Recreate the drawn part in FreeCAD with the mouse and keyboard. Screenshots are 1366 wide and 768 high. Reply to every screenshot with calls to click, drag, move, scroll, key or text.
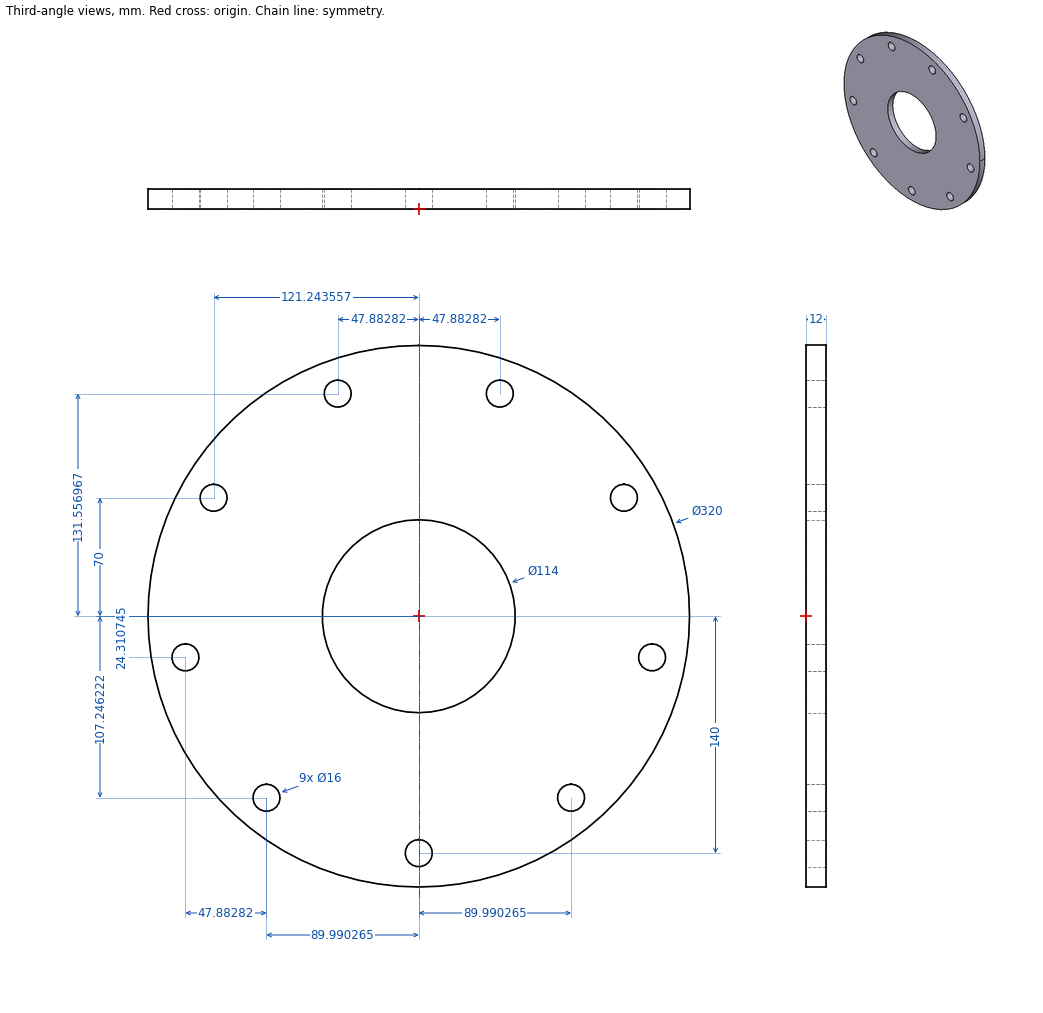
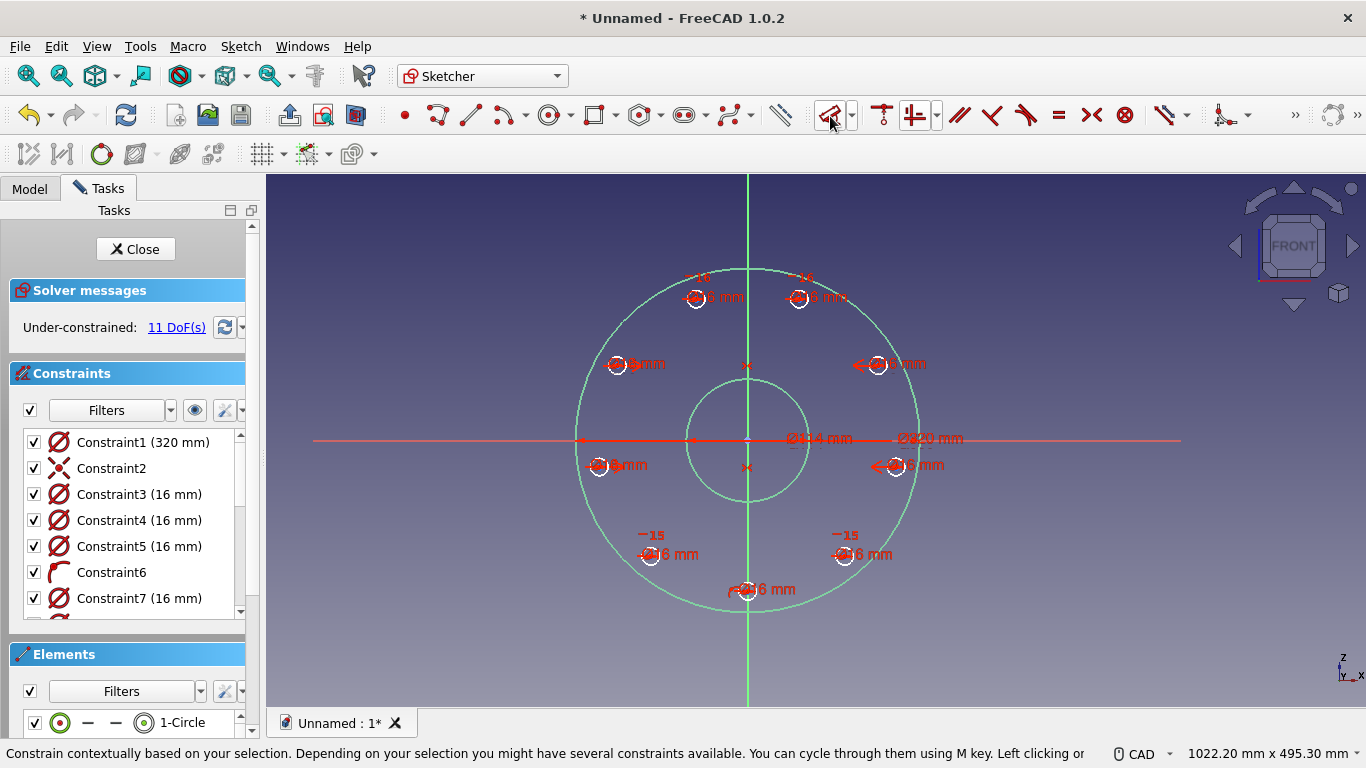
click(617, 366)
click(782, 420)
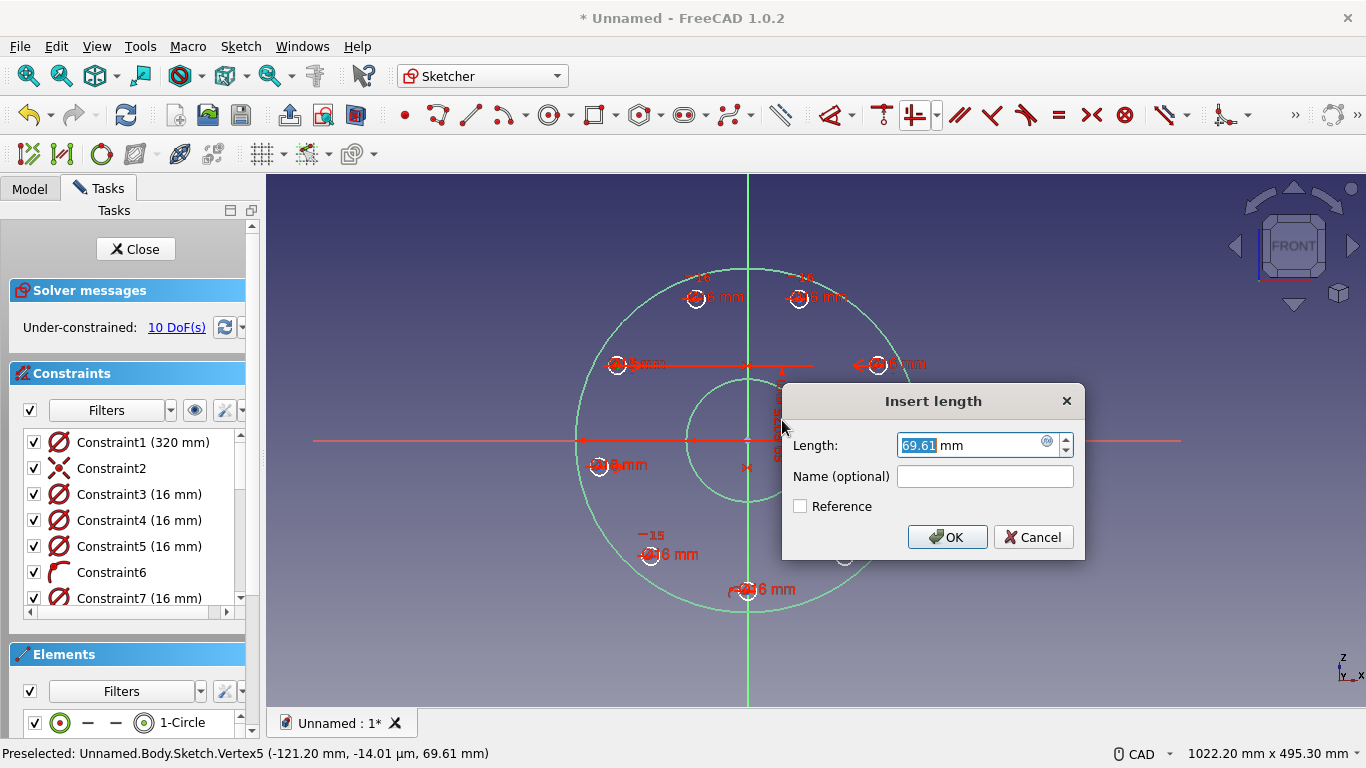
text(70)
key(Return)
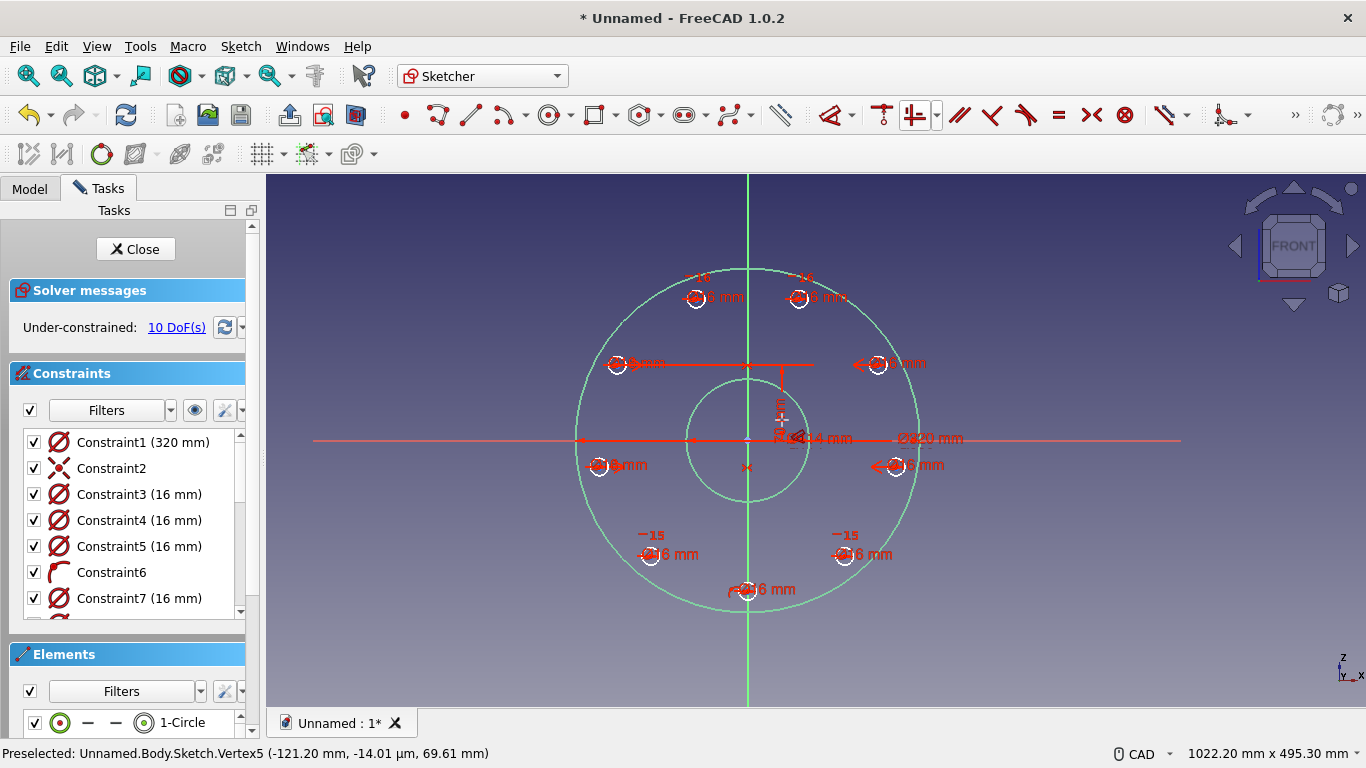
click(748, 591)
click(782, 516)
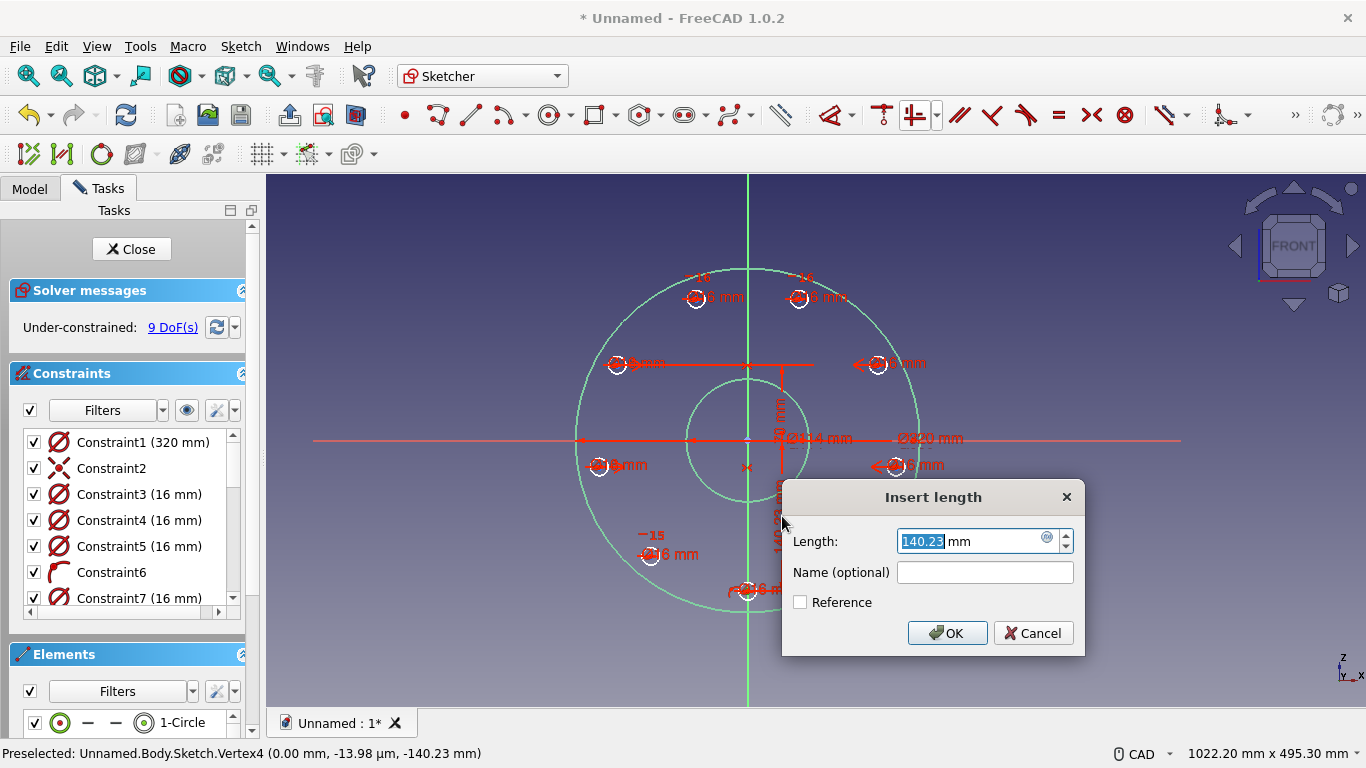
text(140)
key(Return)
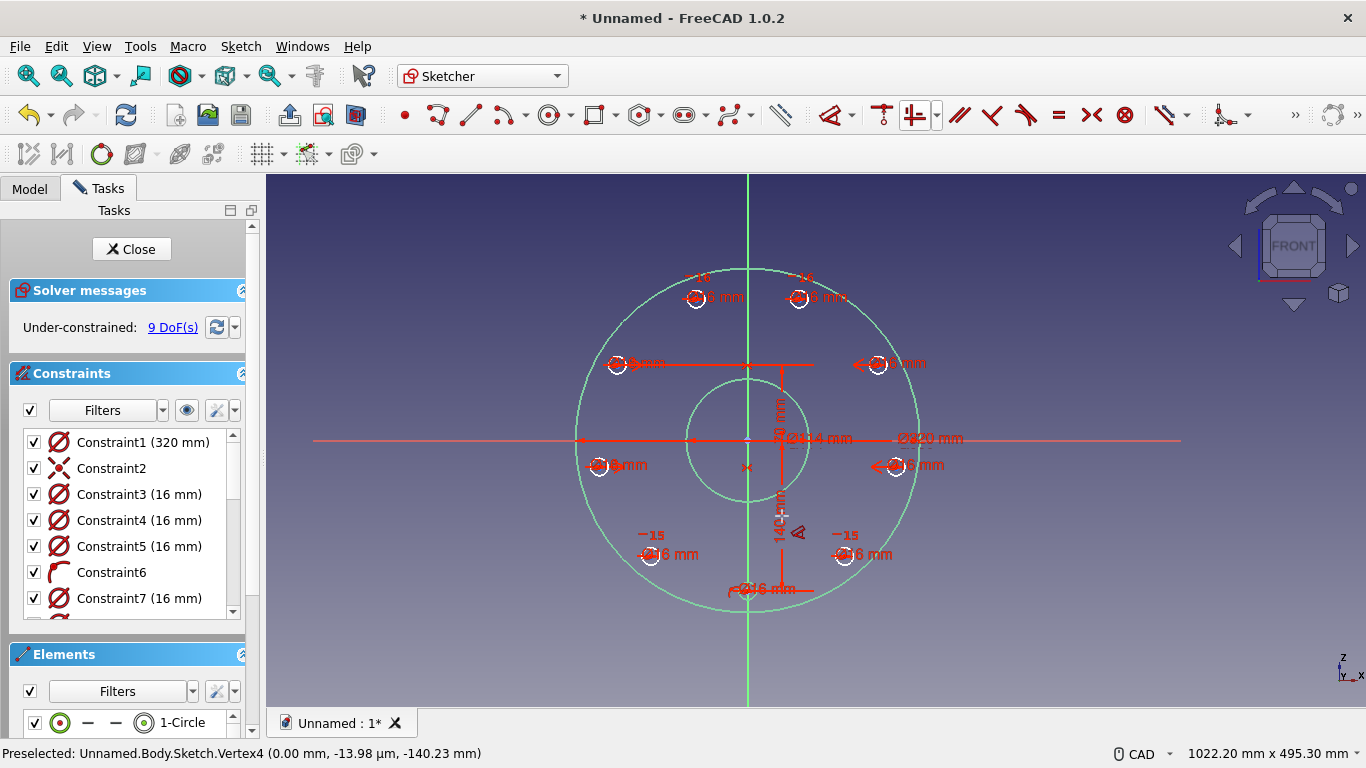
click(696, 299)
click(722, 474)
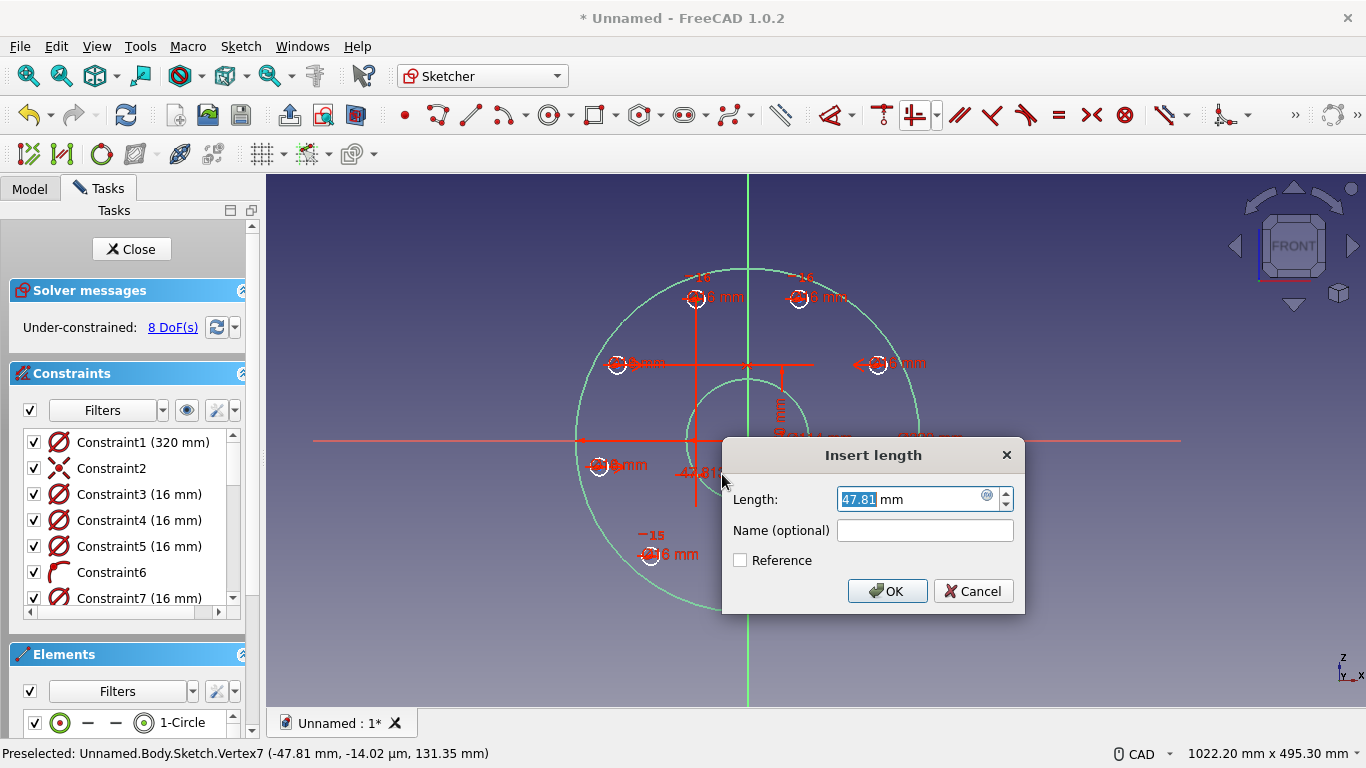
text(47.88282)
key(Return)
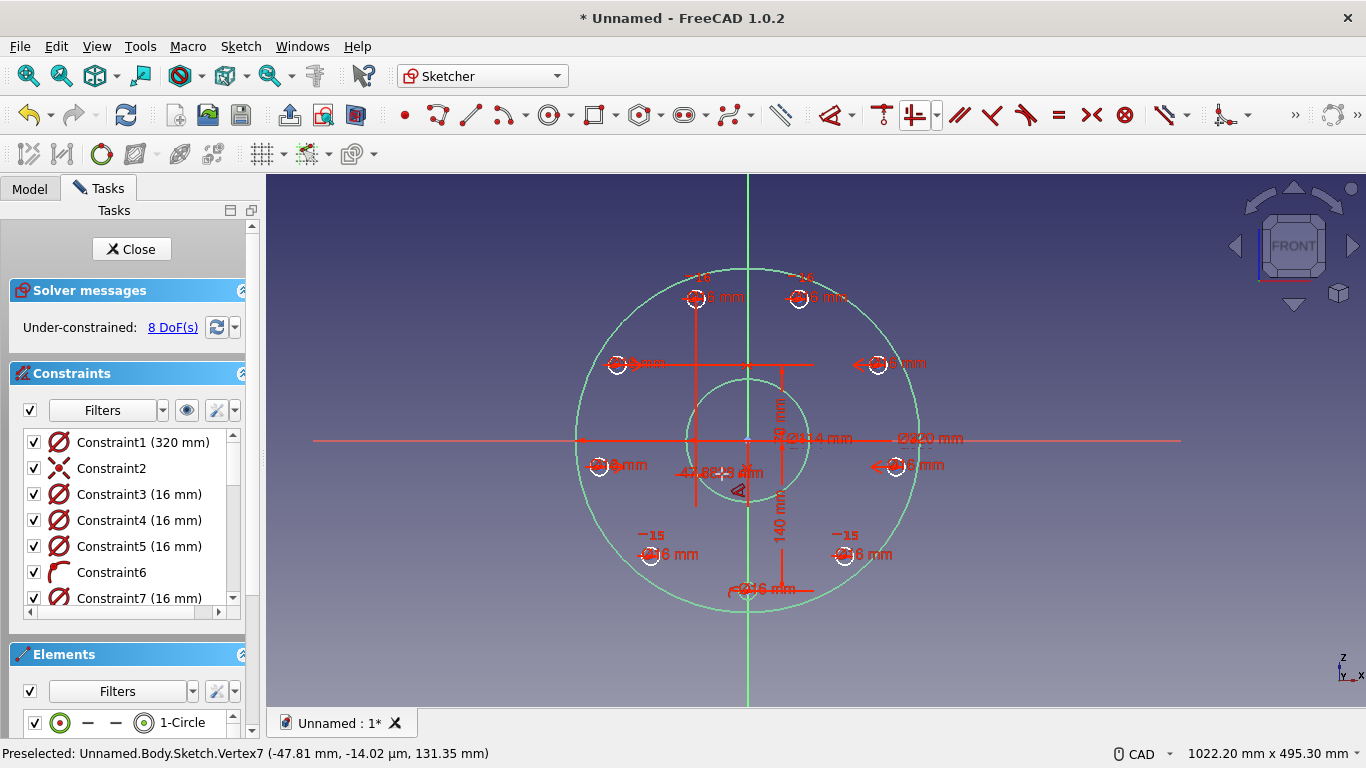
click(799, 299)
click(774, 241)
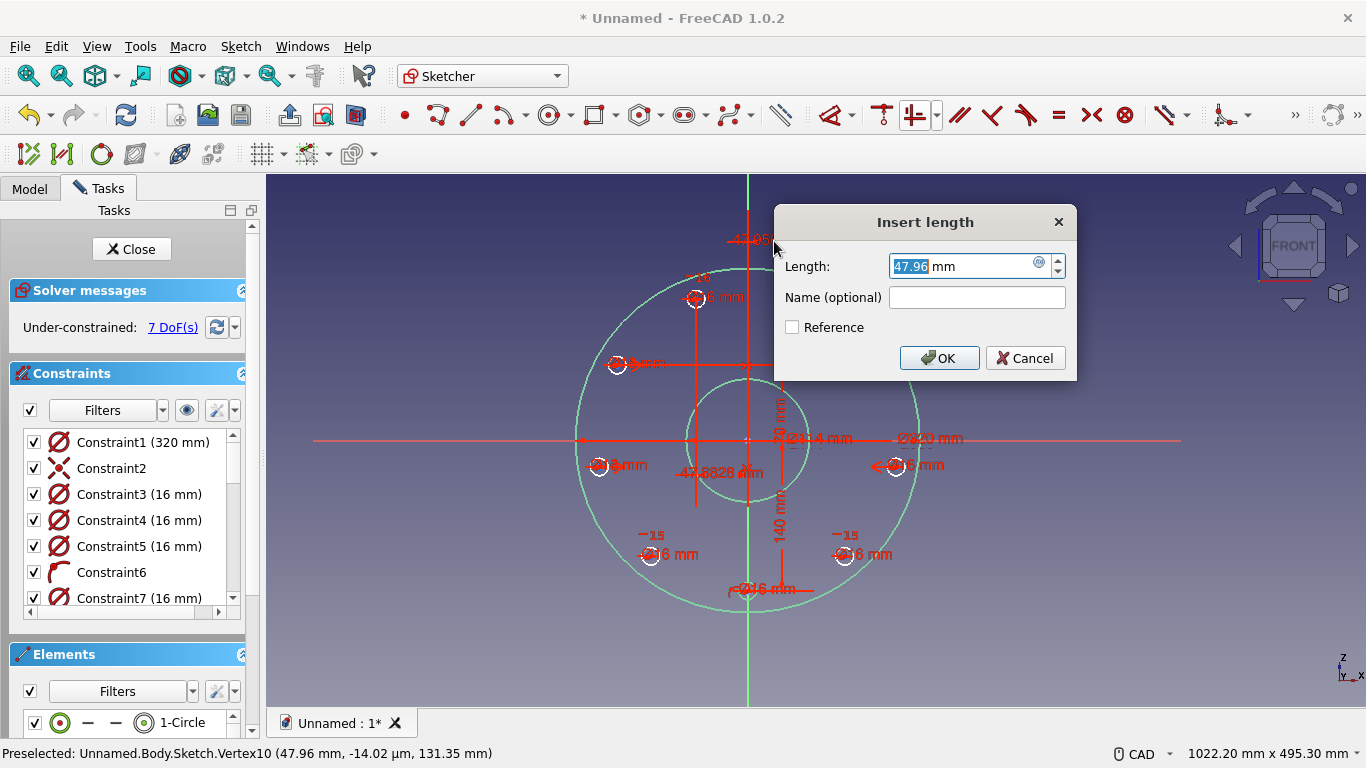
text(47.88282)
key(Return)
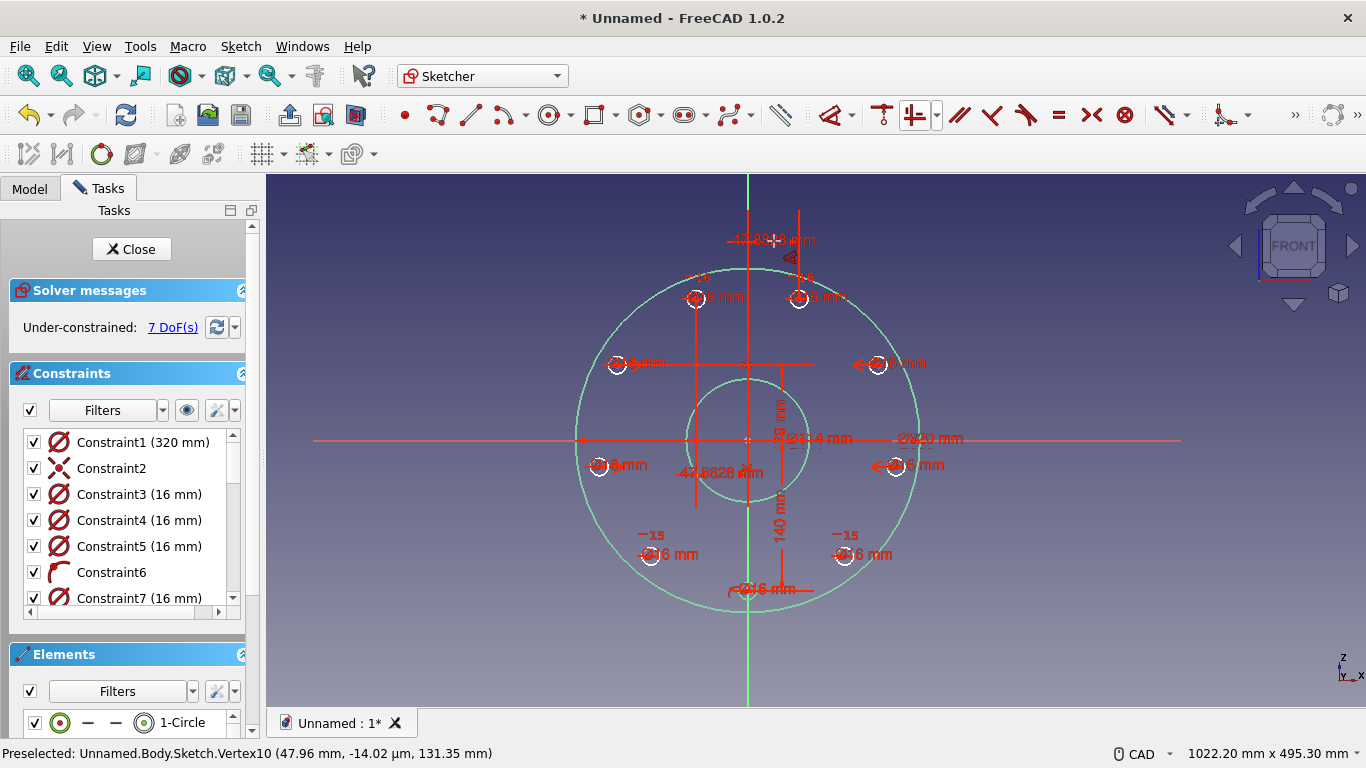
click(651, 556)
click(699, 590)